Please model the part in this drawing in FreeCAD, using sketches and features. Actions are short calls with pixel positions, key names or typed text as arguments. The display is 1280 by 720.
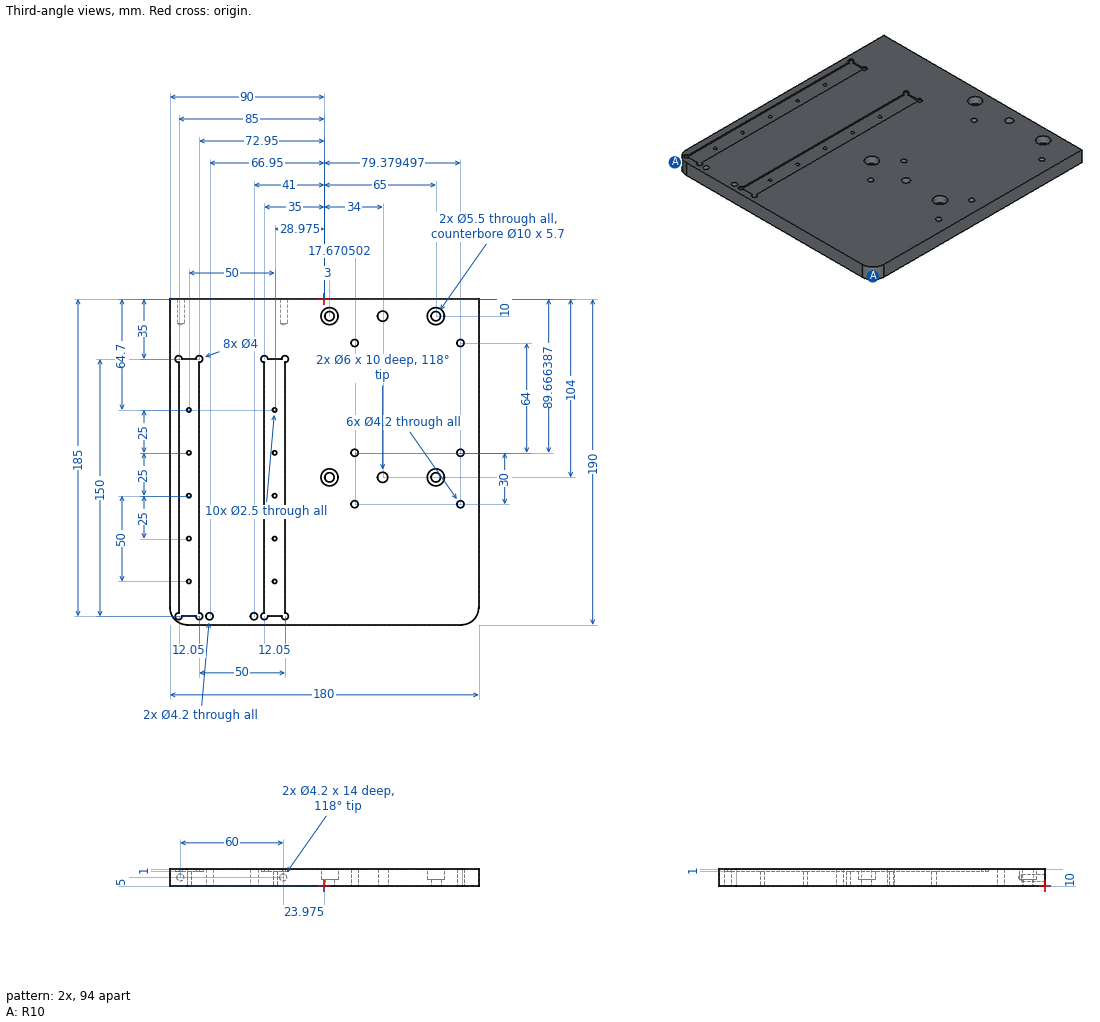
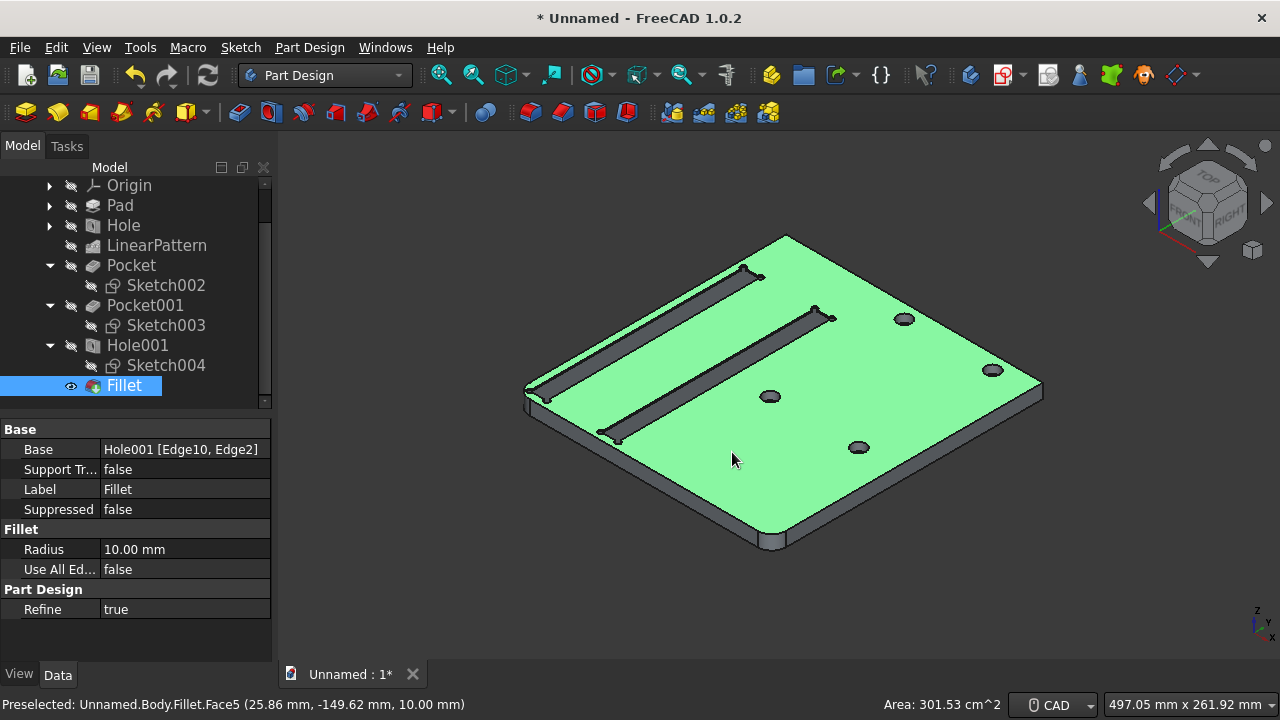
click(1004, 76)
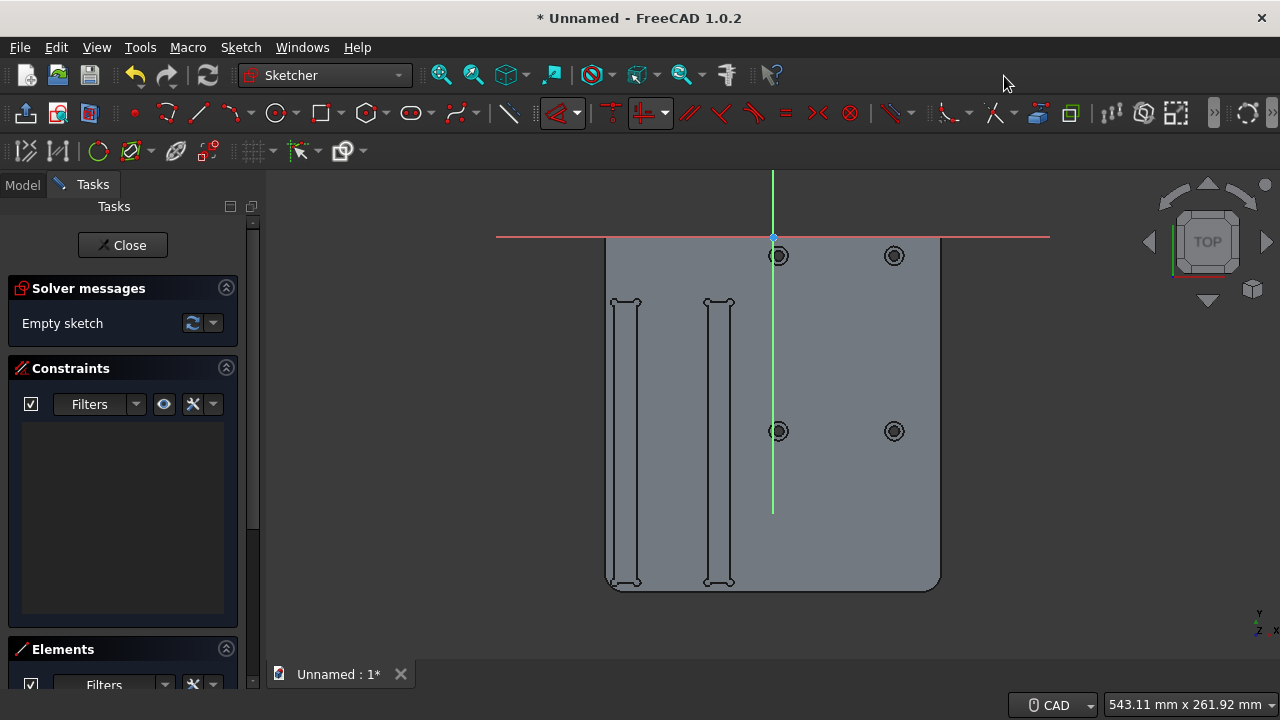
scroll(669, 599, up, 12)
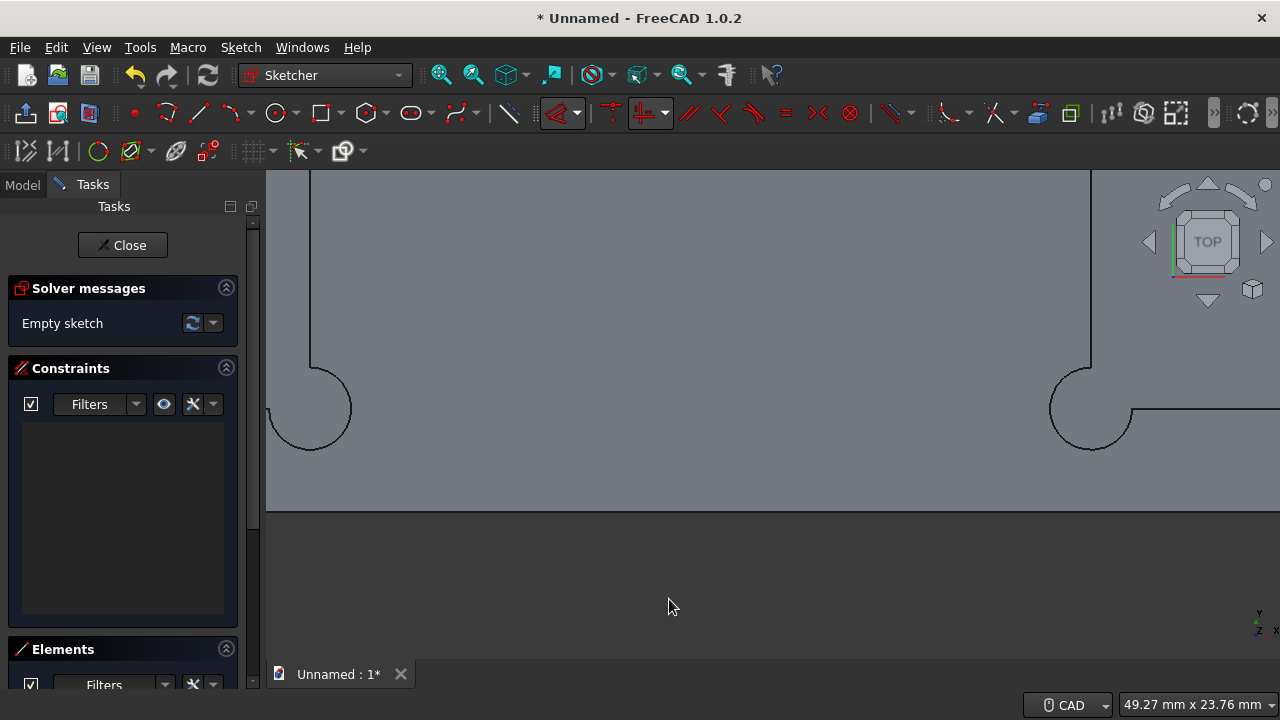
key(g)
key(c)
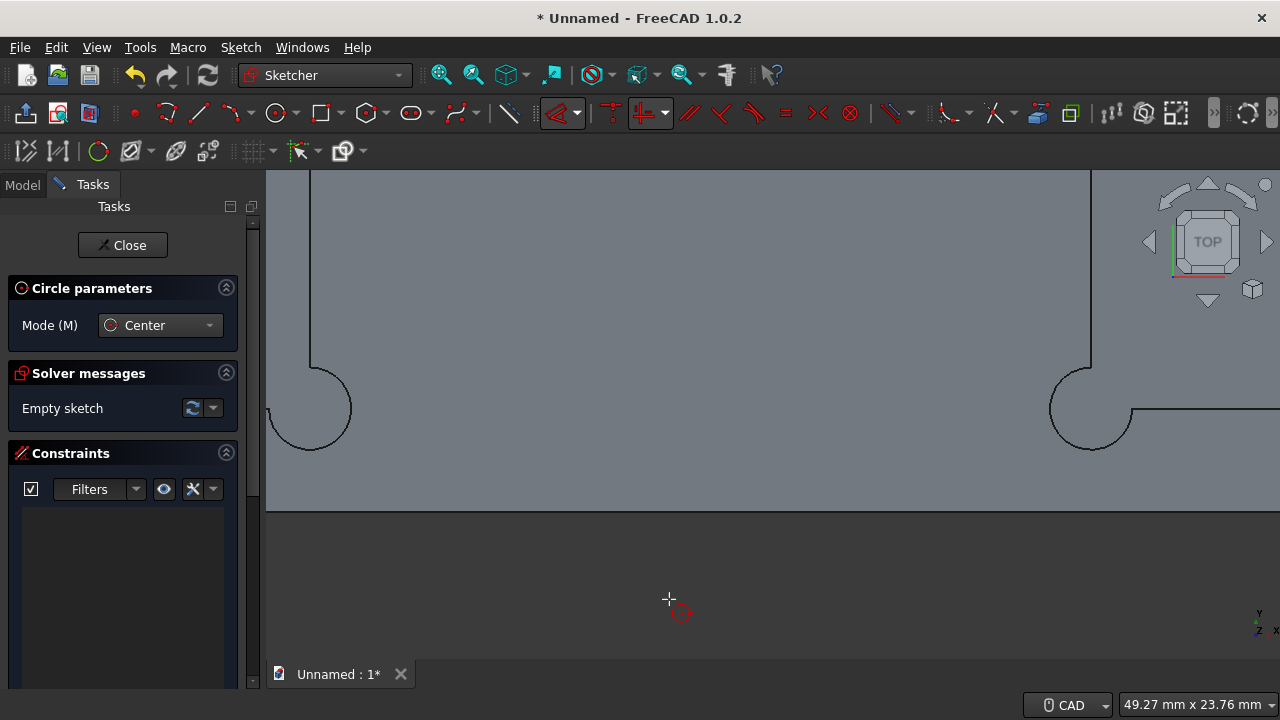
click(434, 409)
move(464, 378)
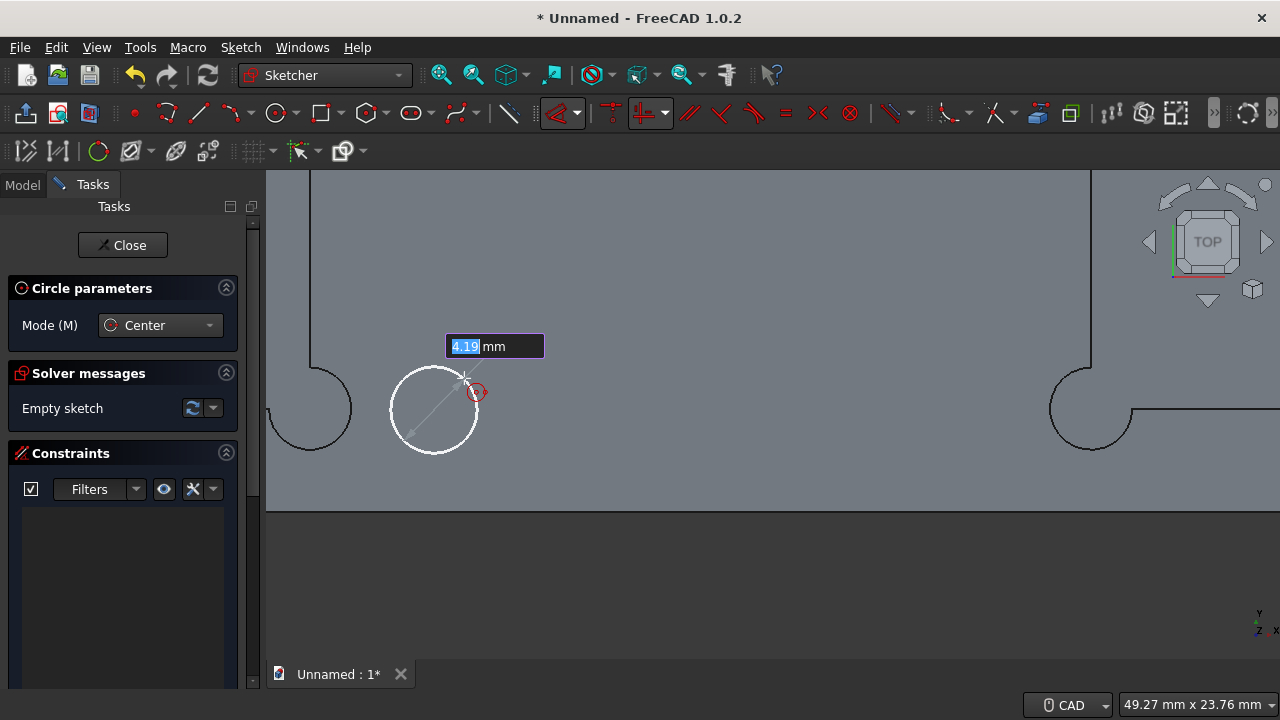
text(4.2)
key(Return)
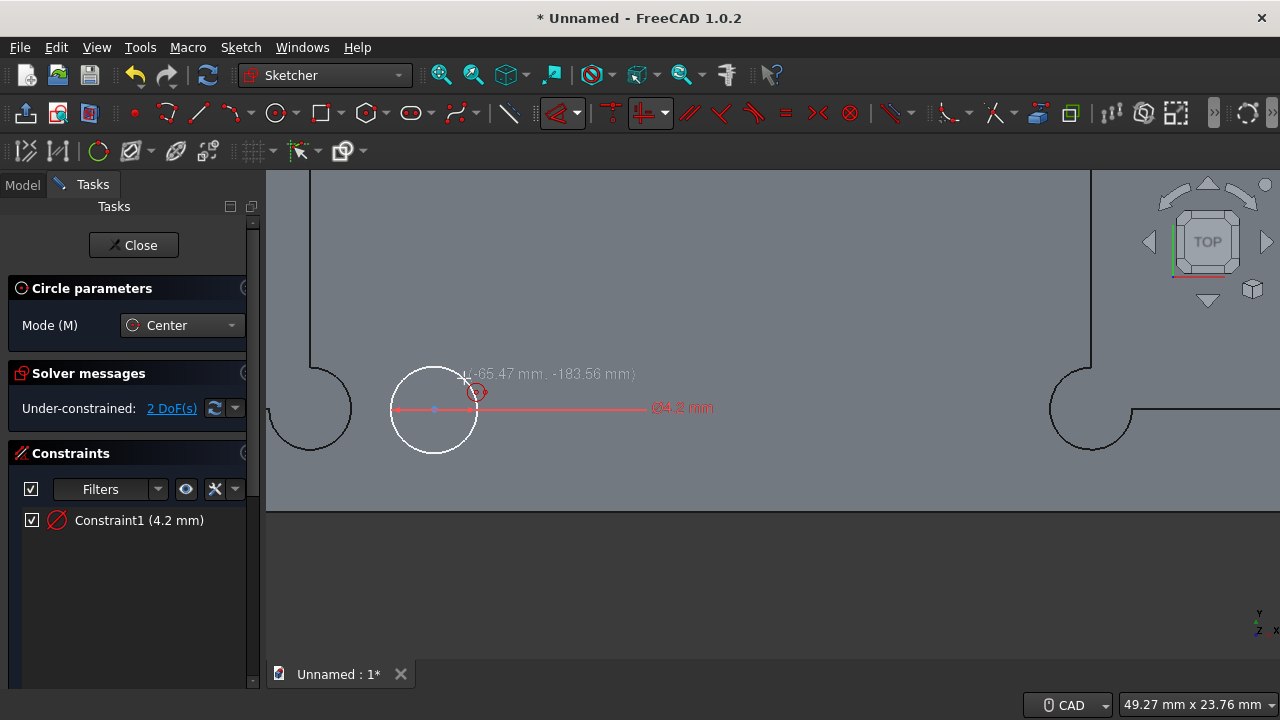
click(968, 409)
move(998, 378)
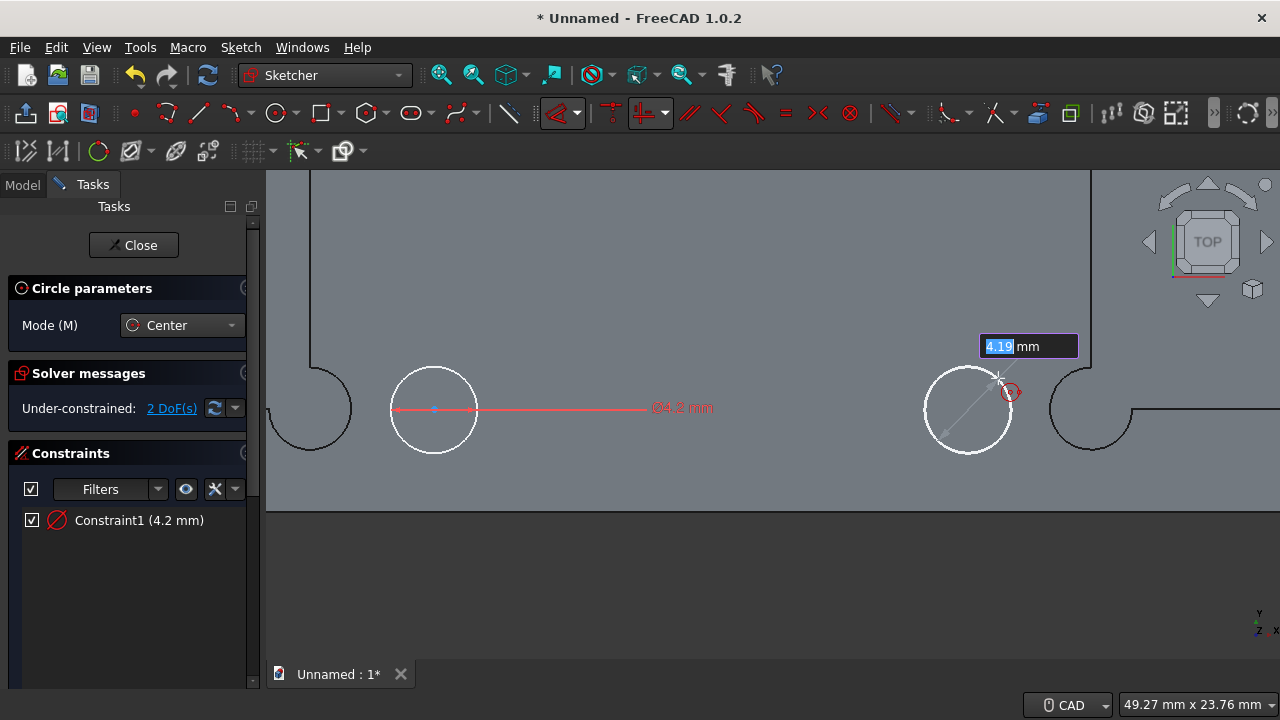
text(4.2)
key(Return)
key(Escape)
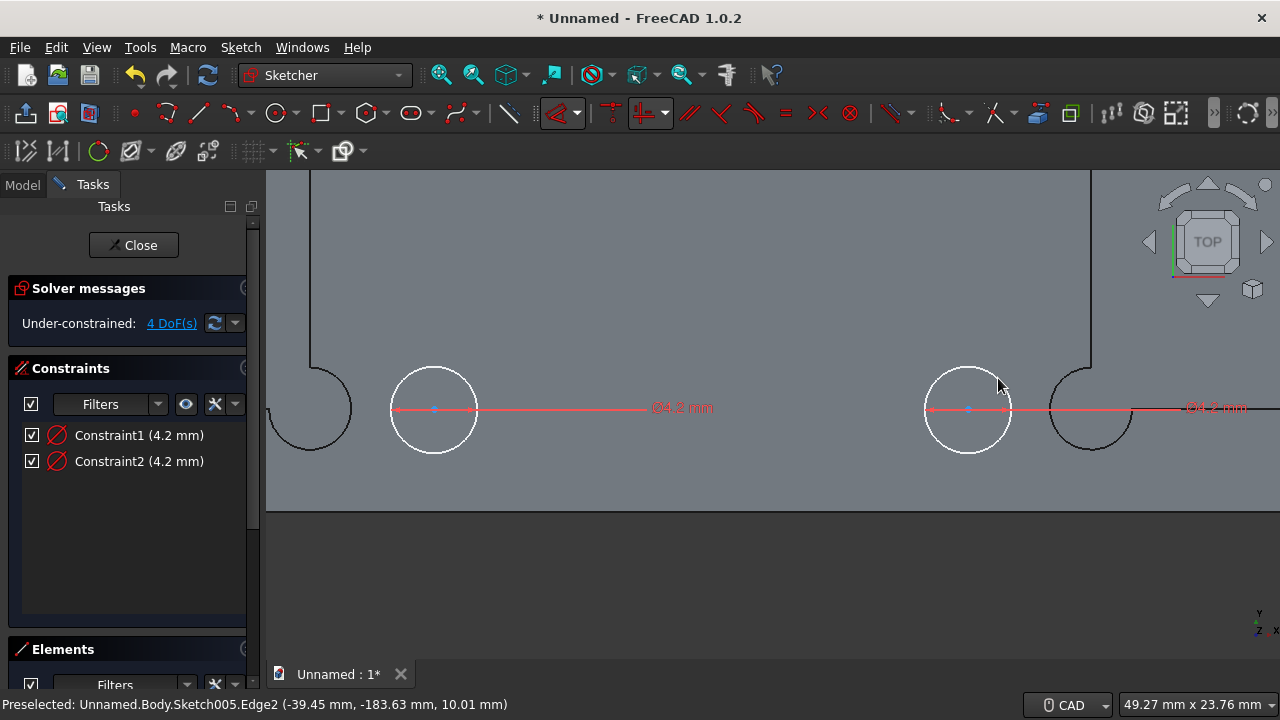
click(434, 410)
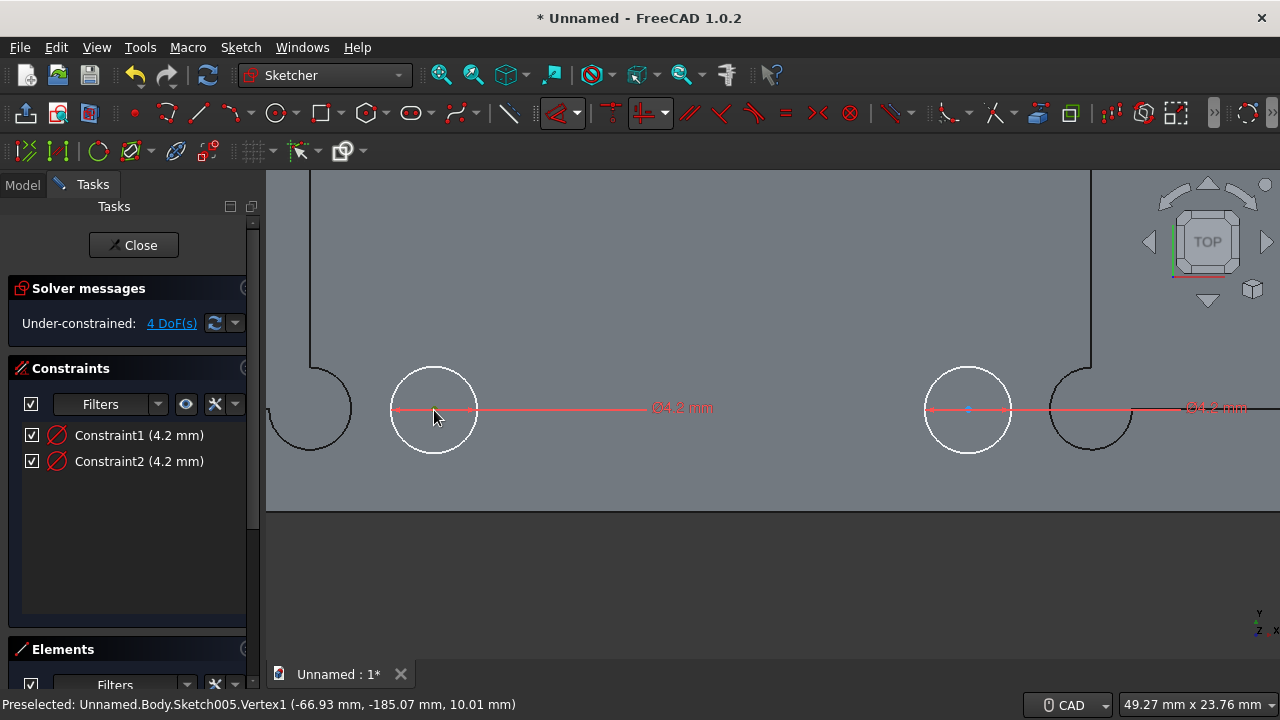
click(968, 410)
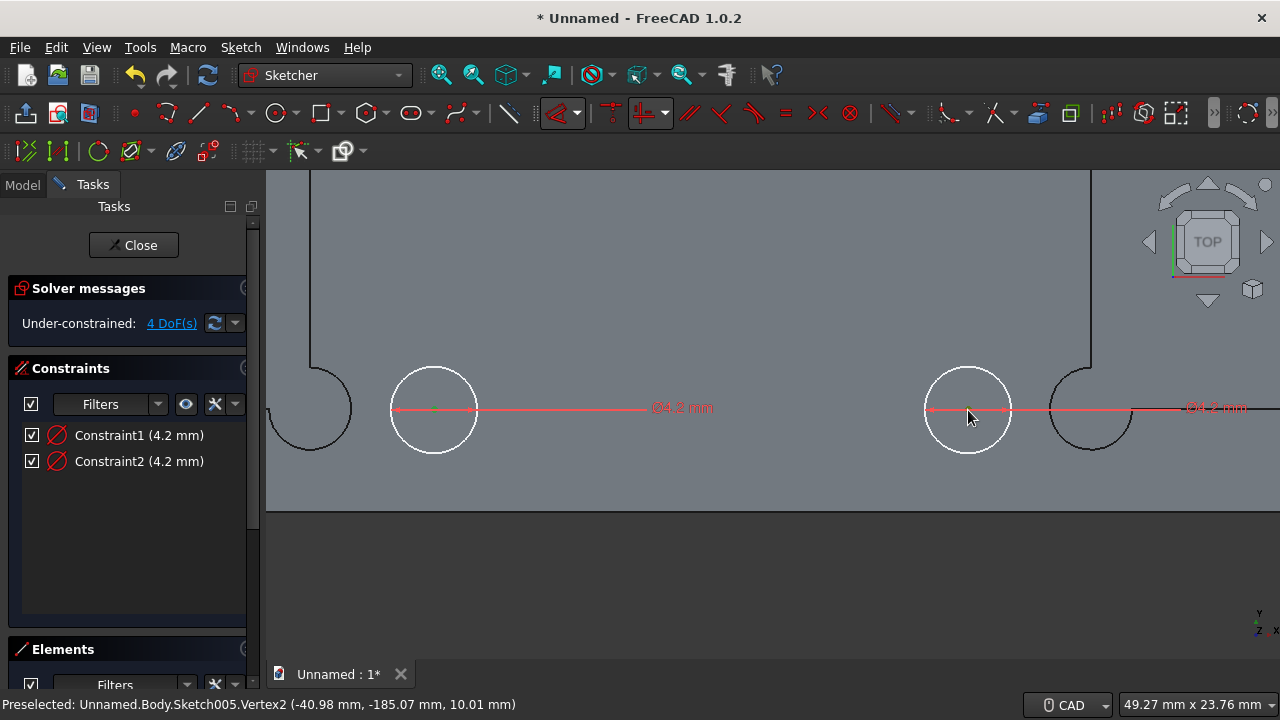
key(h)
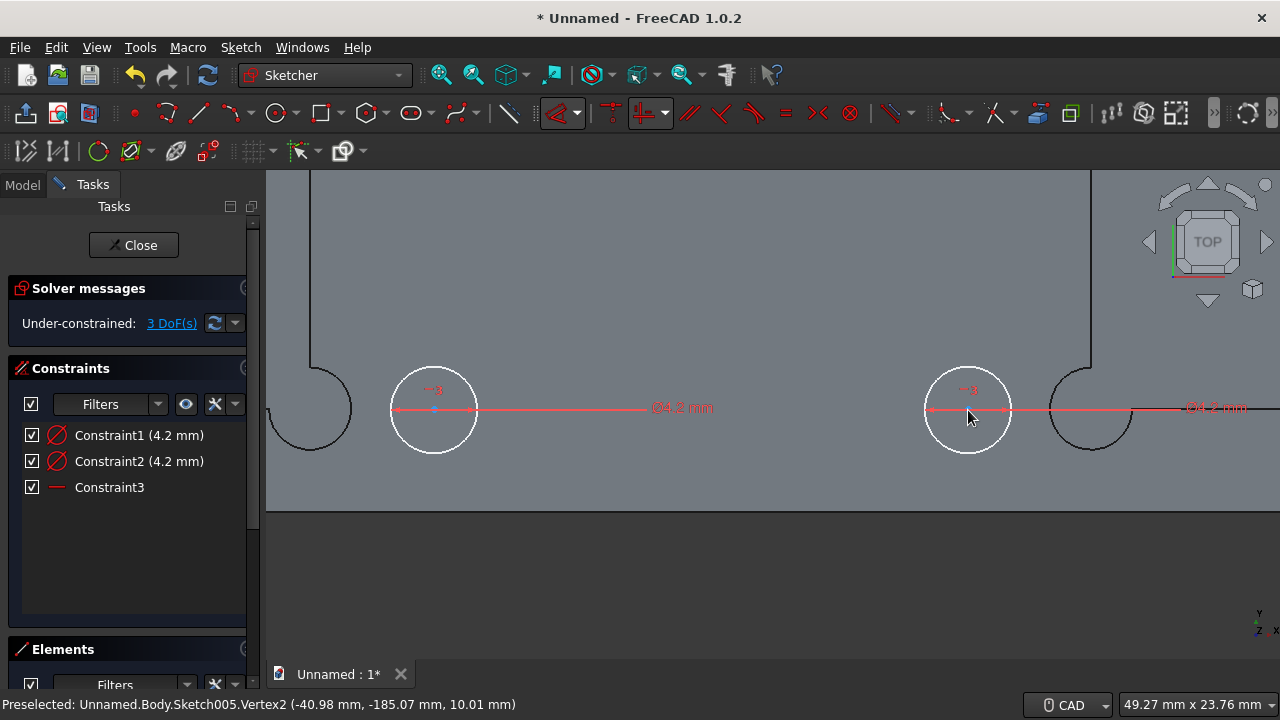
click(968, 410)